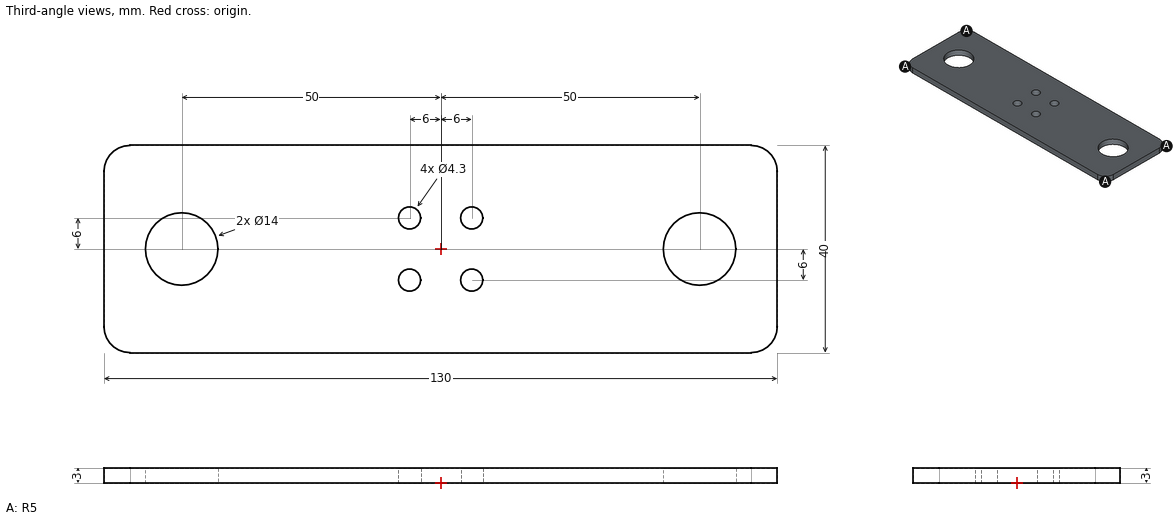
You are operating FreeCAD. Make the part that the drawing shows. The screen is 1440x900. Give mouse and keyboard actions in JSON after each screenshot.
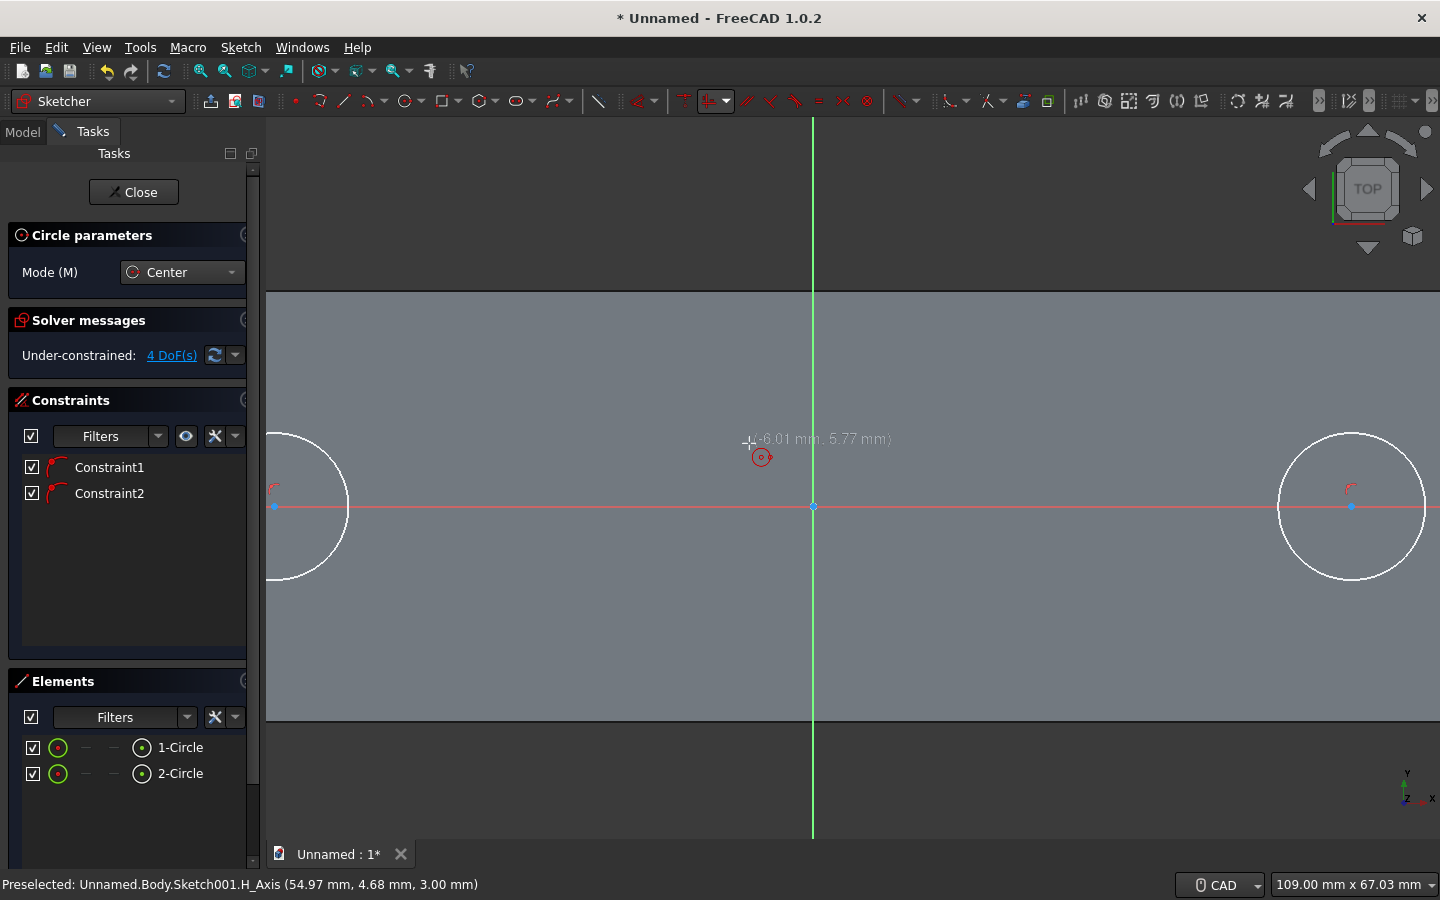
{"action": "left_click", "coordinate": [749, 442]}
{"action": "left_click", "coordinate": [765, 426]}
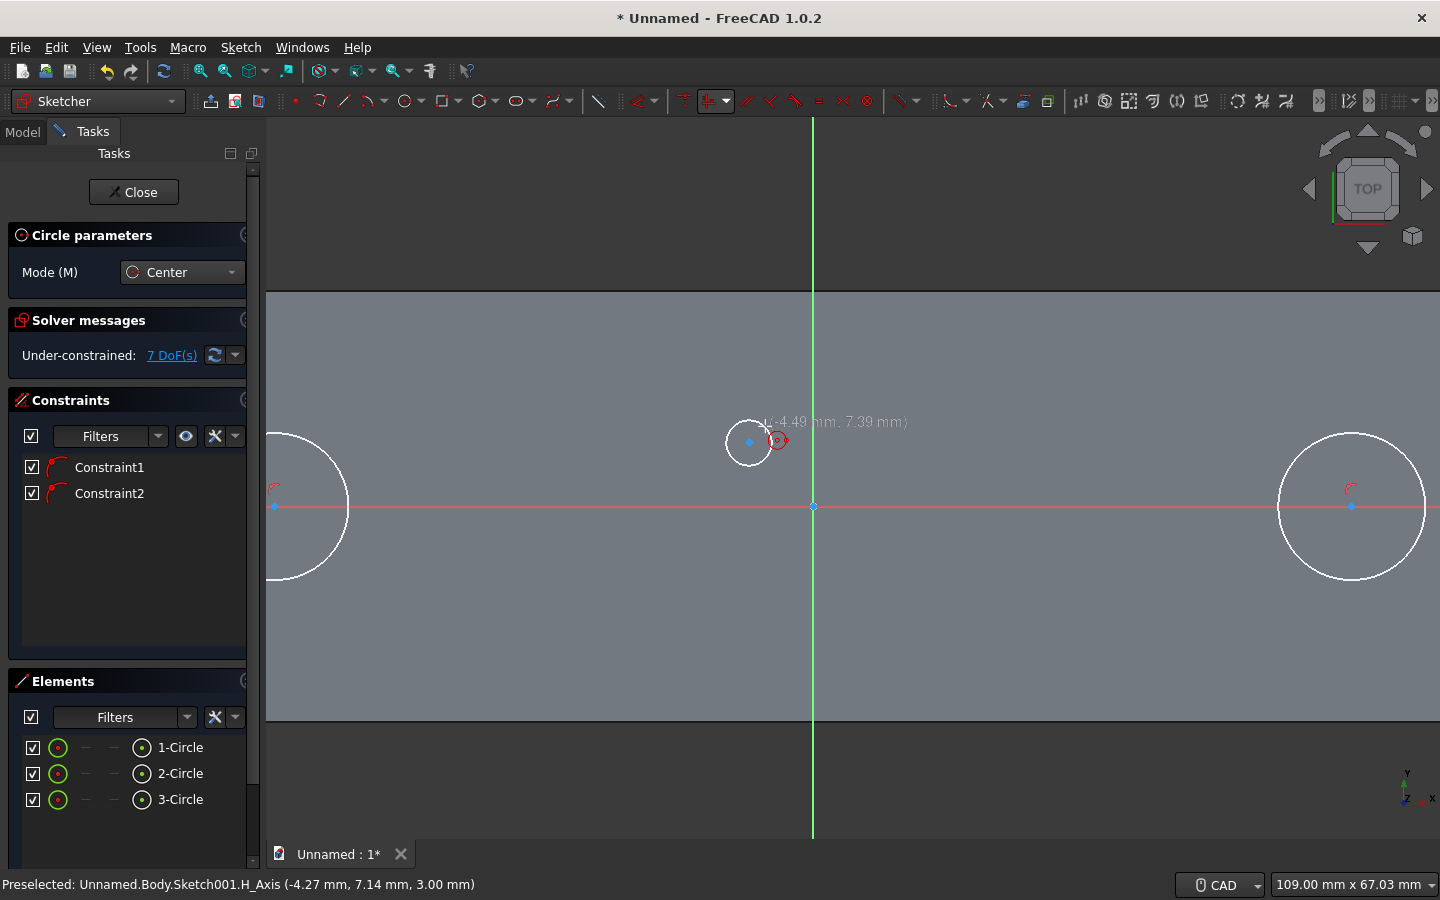
{"action": "left_click", "coordinate": [878, 442]}
{"action": "left_click", "coordinate": [894, 426]}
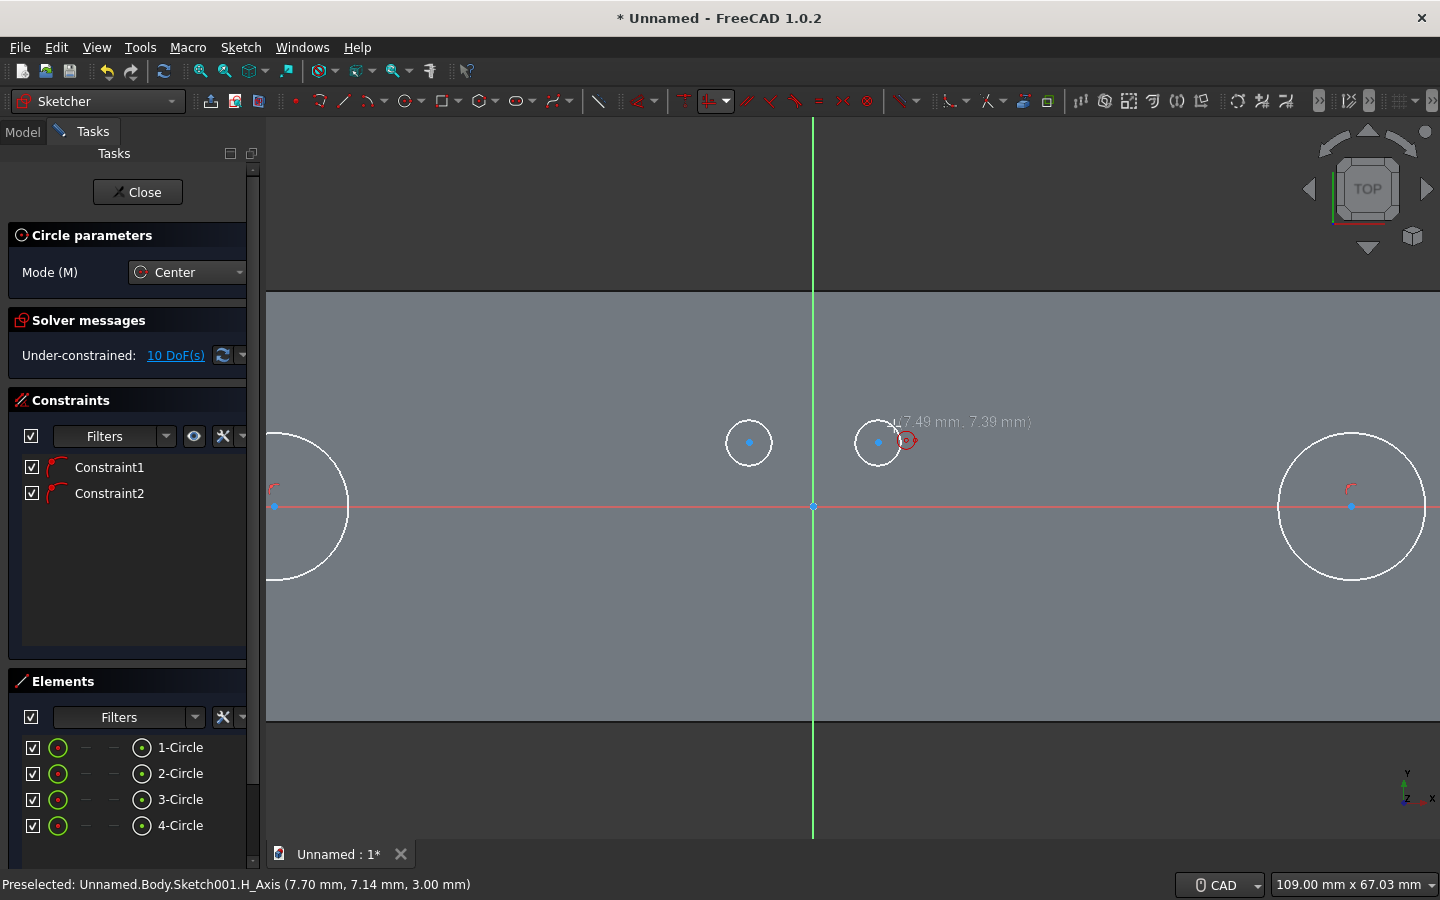
{"action": "left_click", "coordinate": [878, 571]}
{"action": "left_click", "coordinate": [894, 555]}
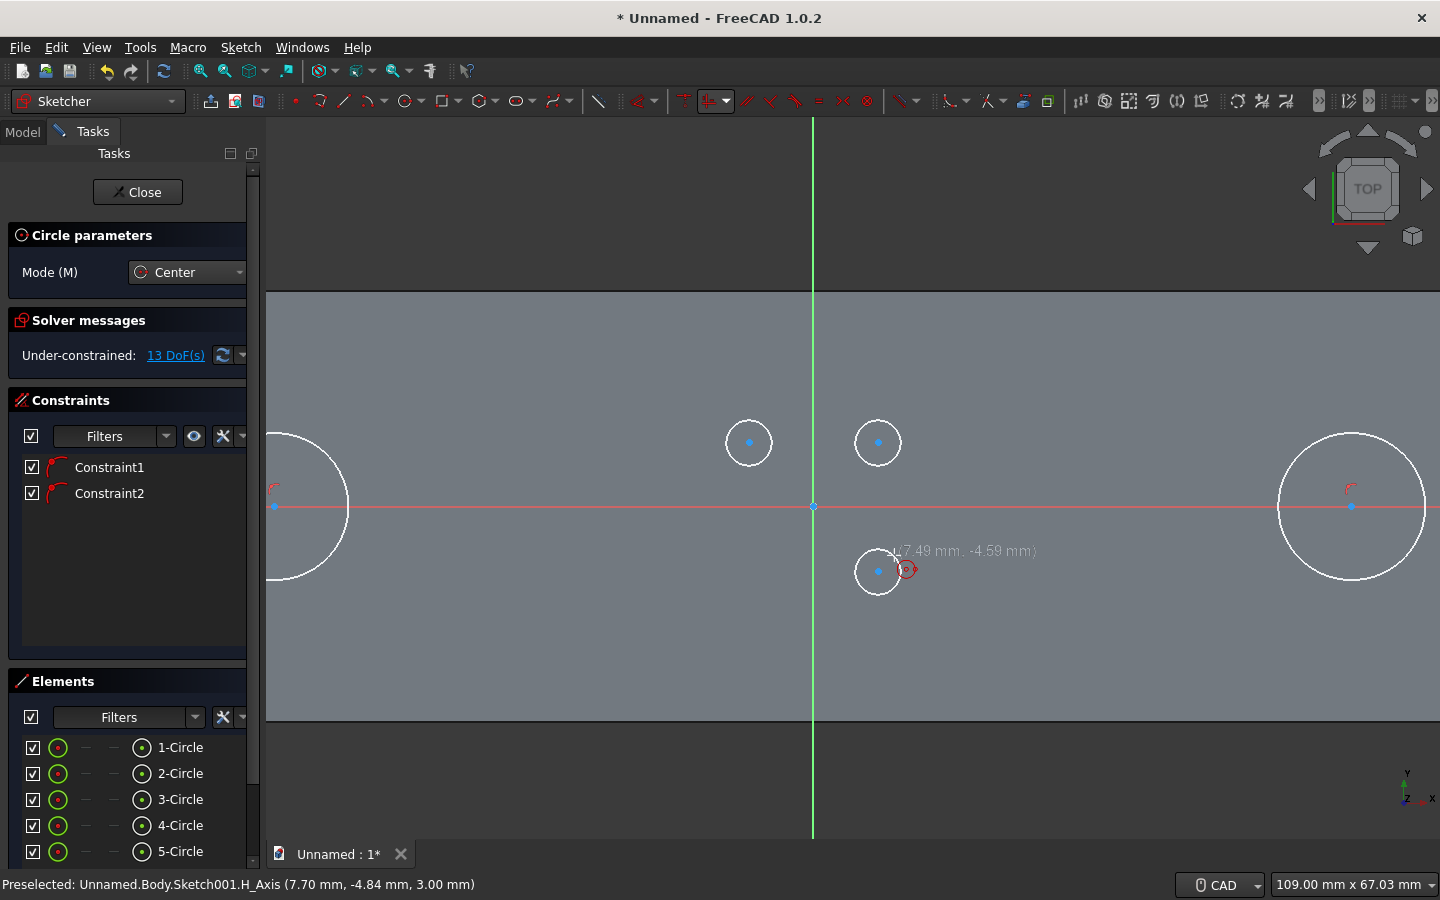
{"action": "left_click", "coordinate": [749, 571]}
{"action": "left_click", "coordinate": [765, 555]}
{"action": "key", "text": "Escape"}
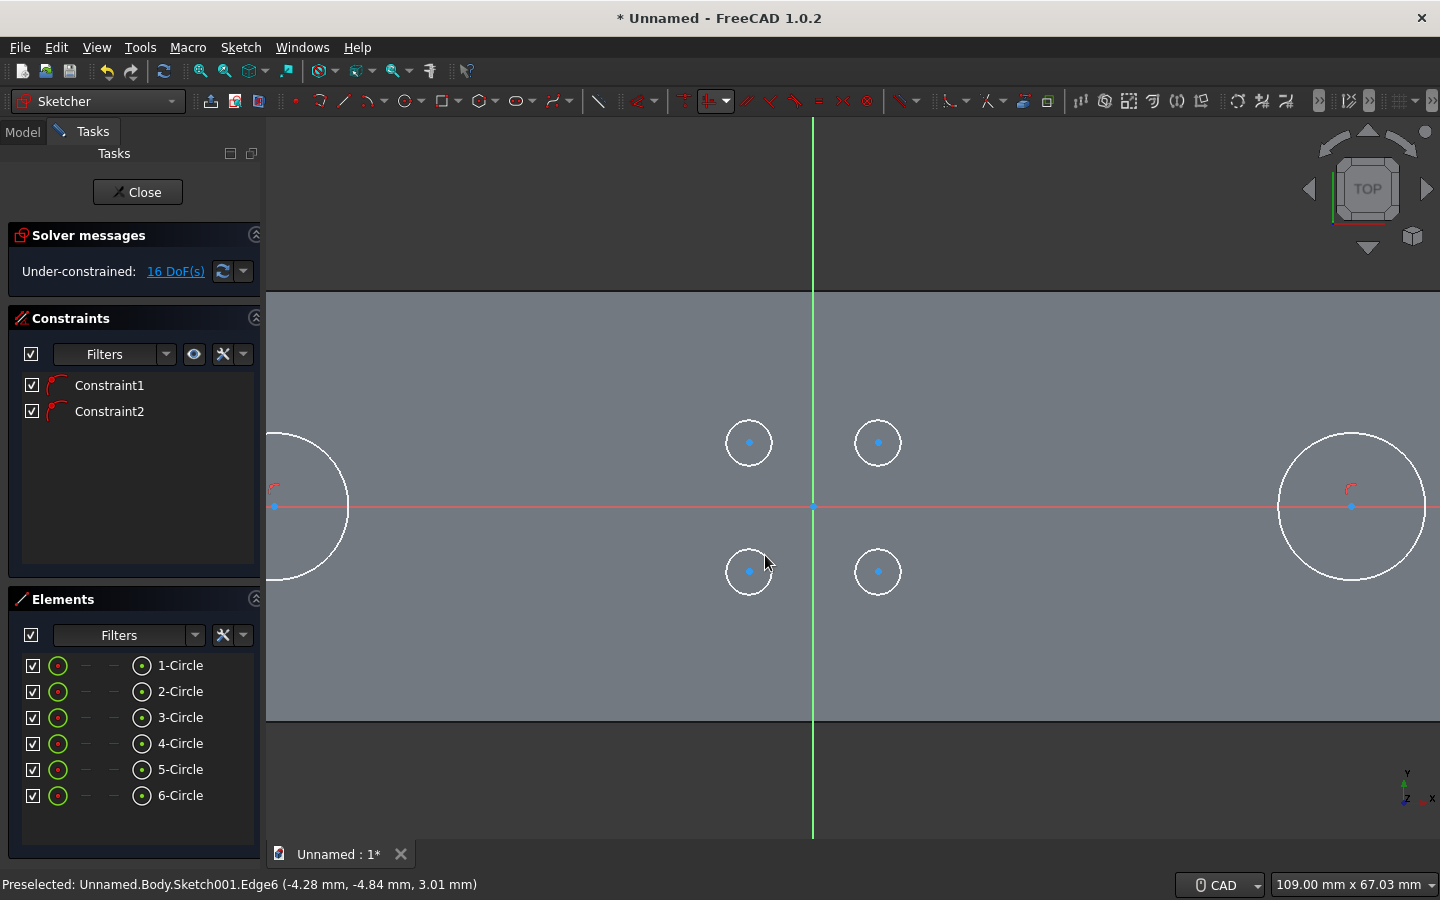
{"action": "left_click", "coordinate": [327, 454]}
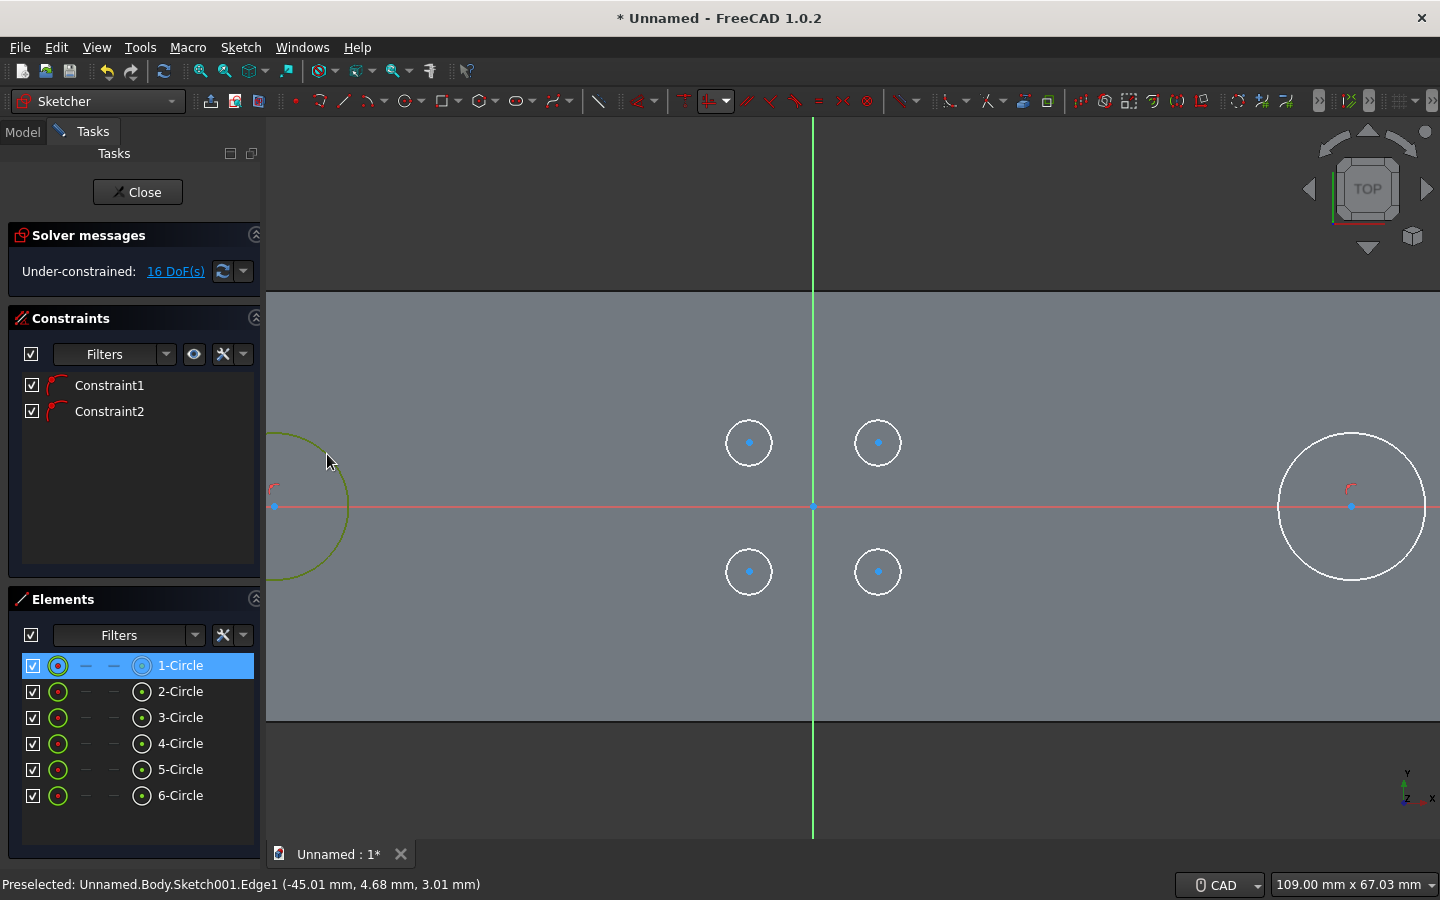
{"action": "scroll", "coordinate": [749, 443], "scroll_direction": "down", "scroll_amount": 3}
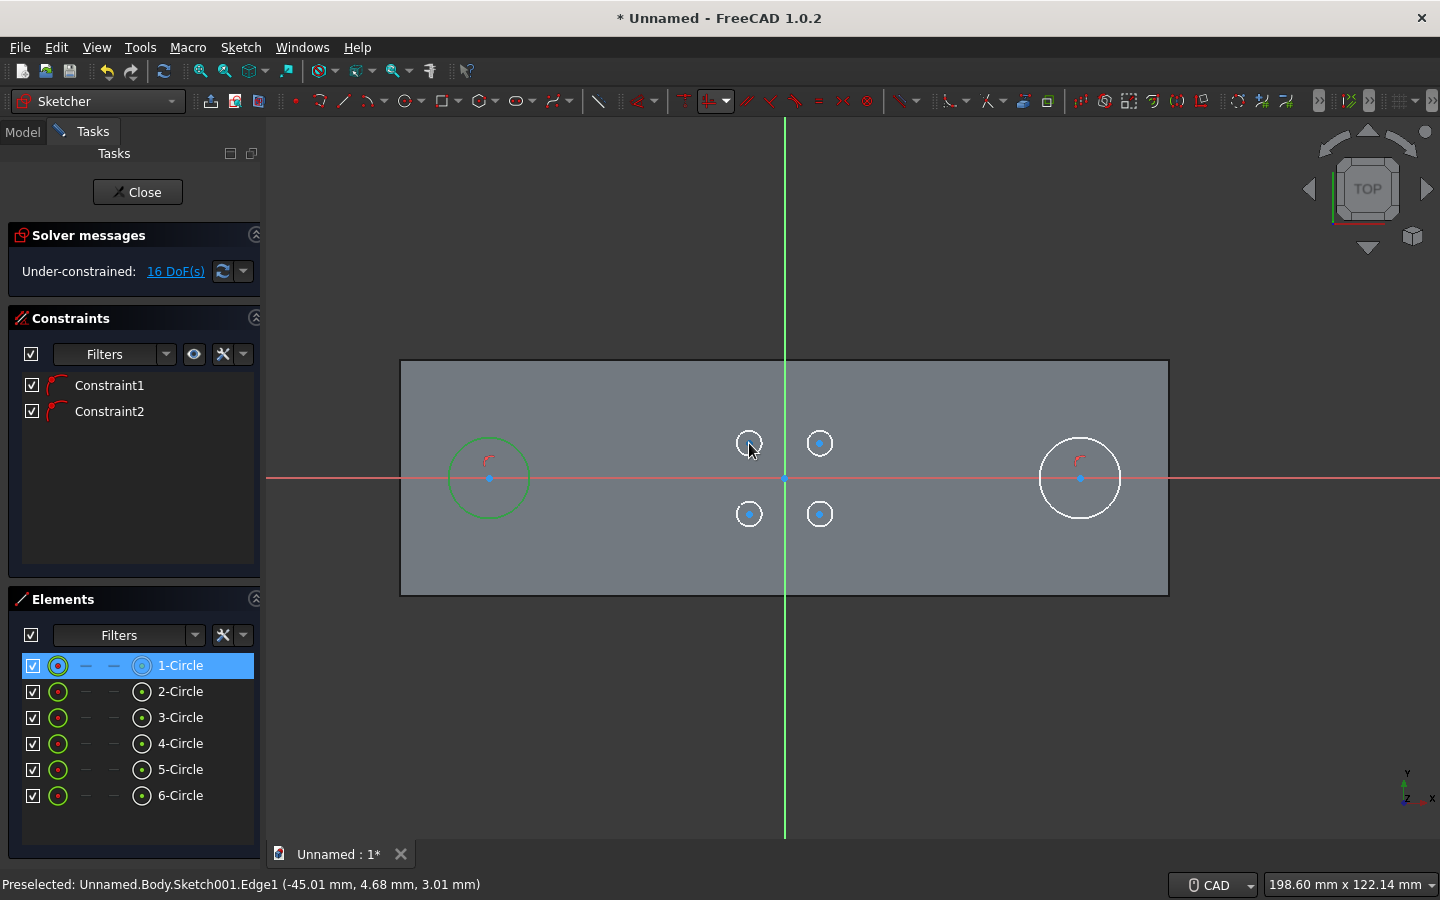
{"action": "left_click", "coordinate": [1108, 449]}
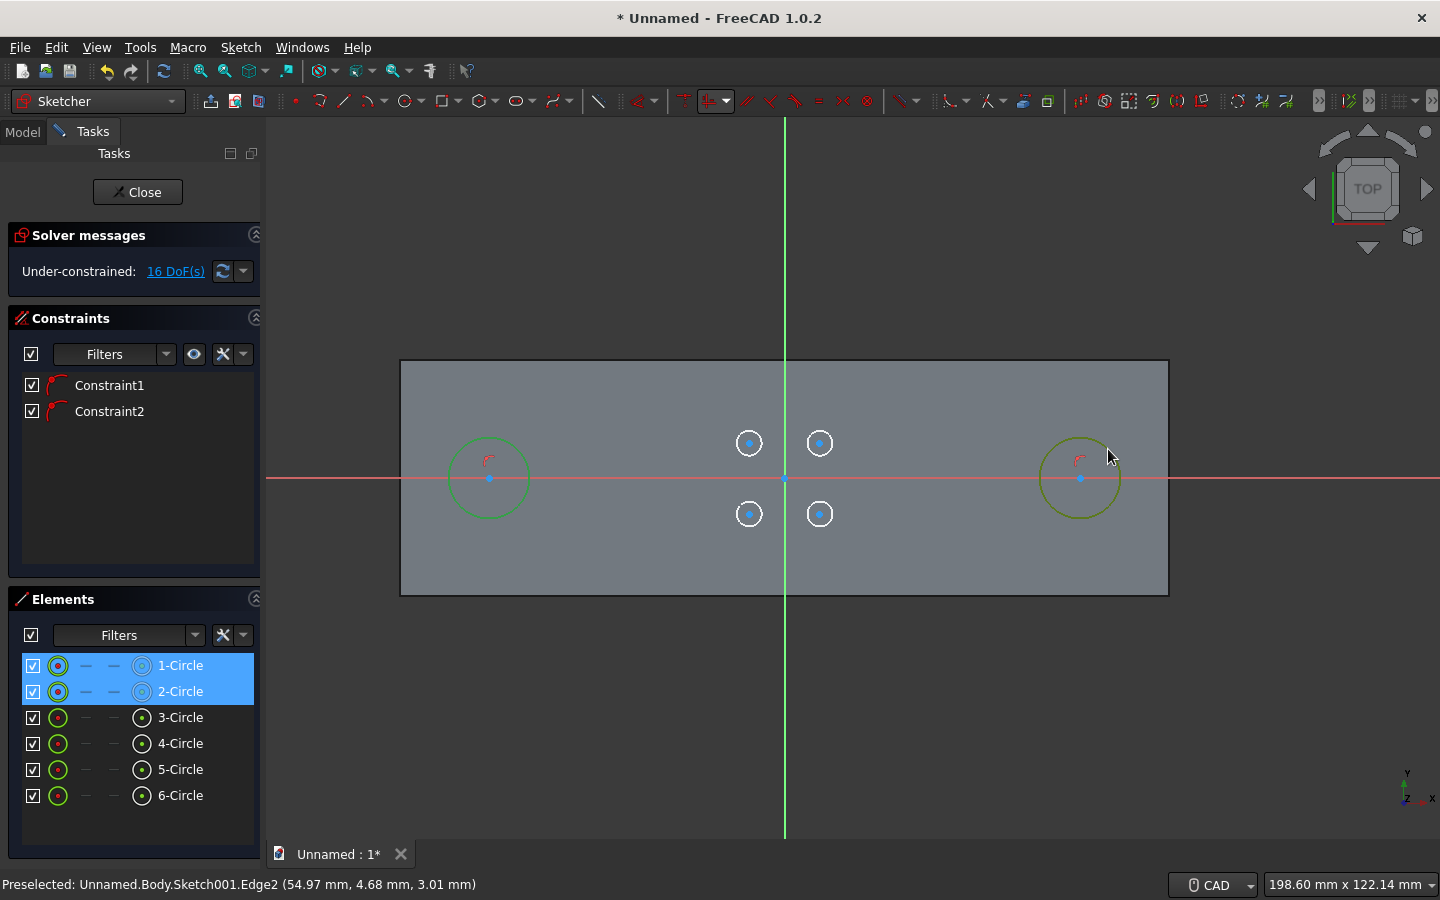
{"action": "key", "text": "e"}